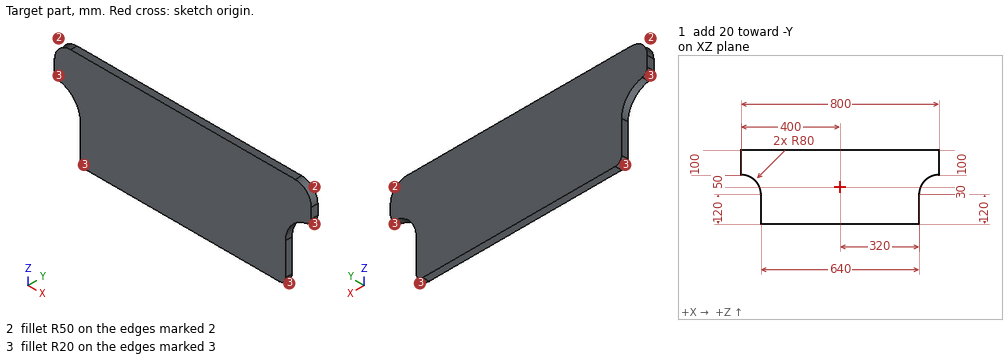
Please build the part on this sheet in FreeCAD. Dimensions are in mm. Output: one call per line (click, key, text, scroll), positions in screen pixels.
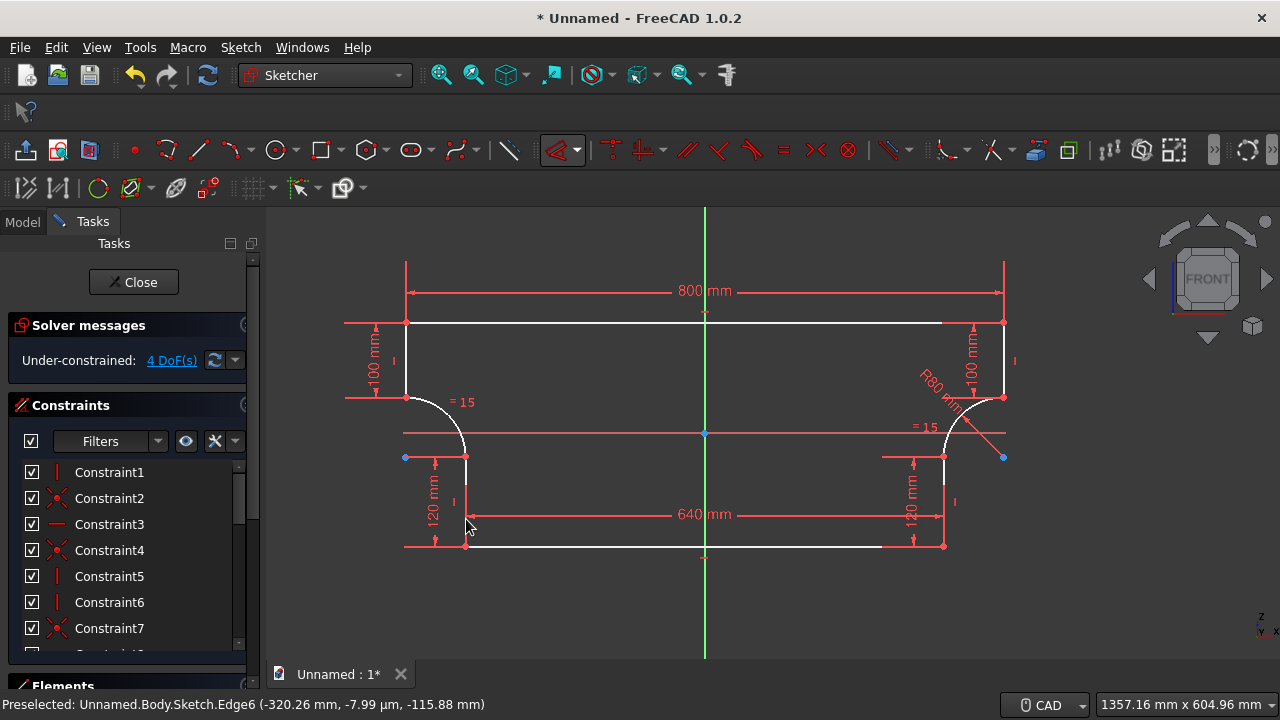
click(406, 398)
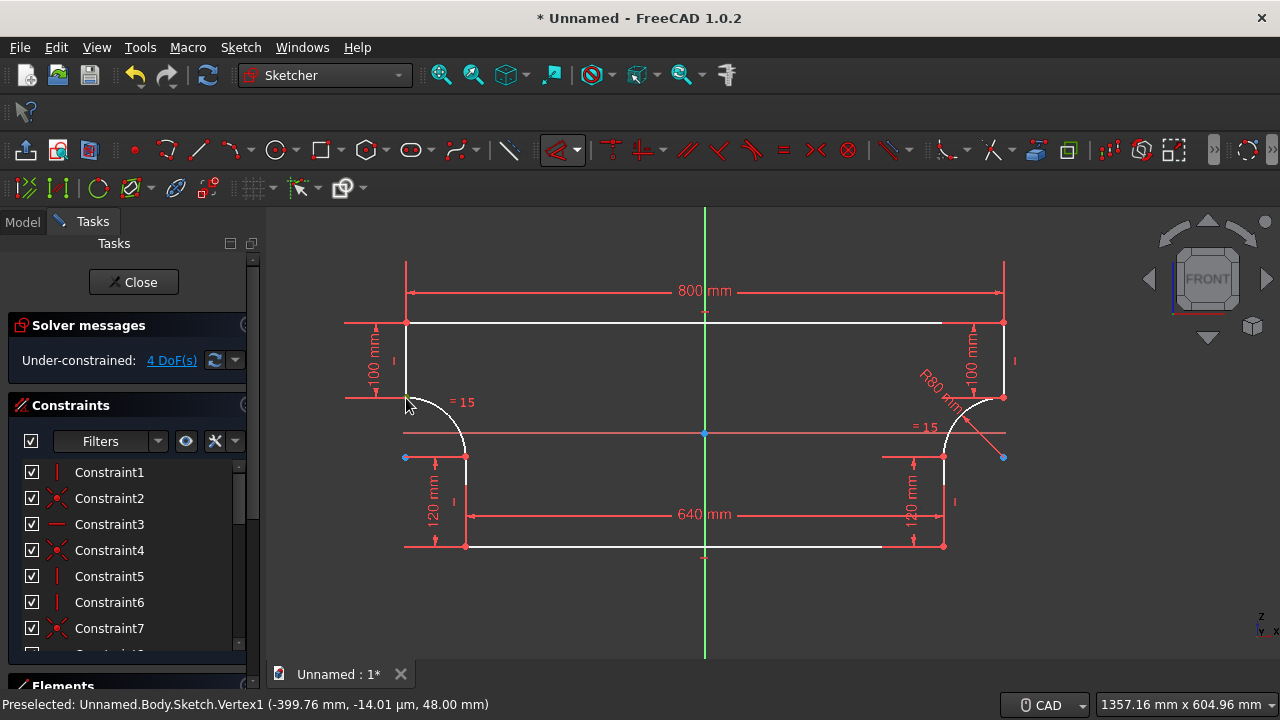
key(i)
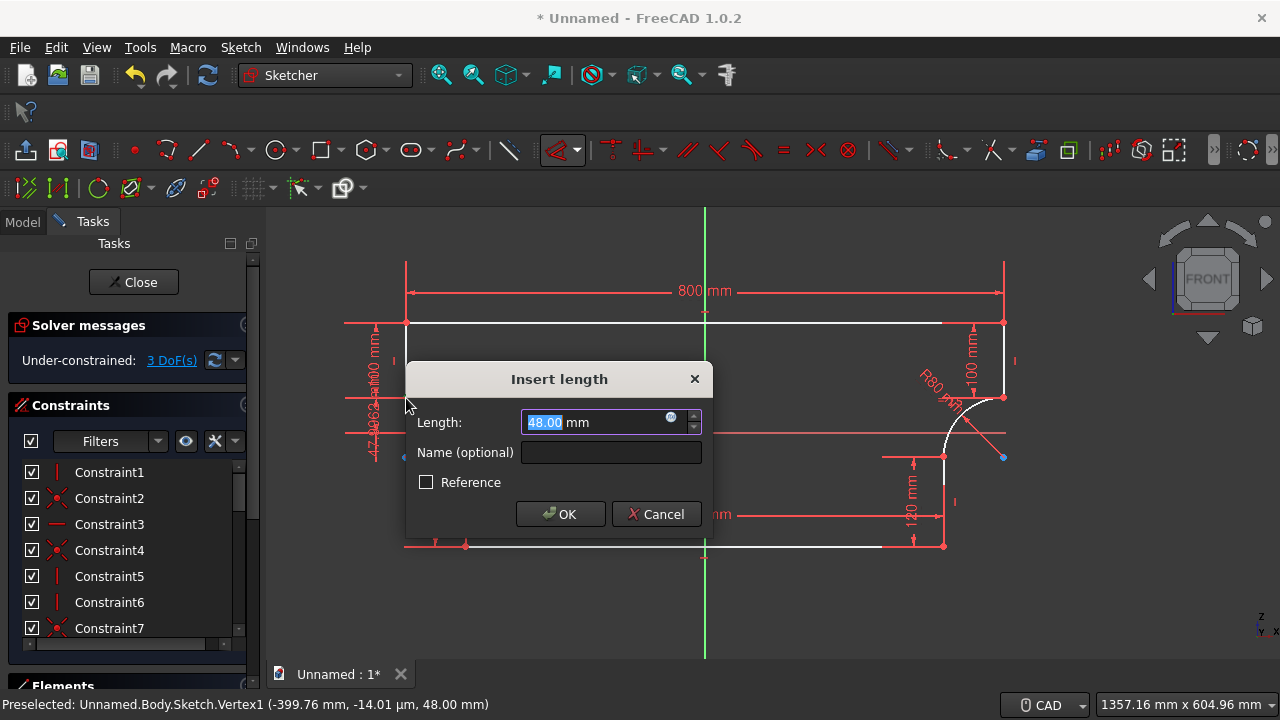
text(50)
key(Return)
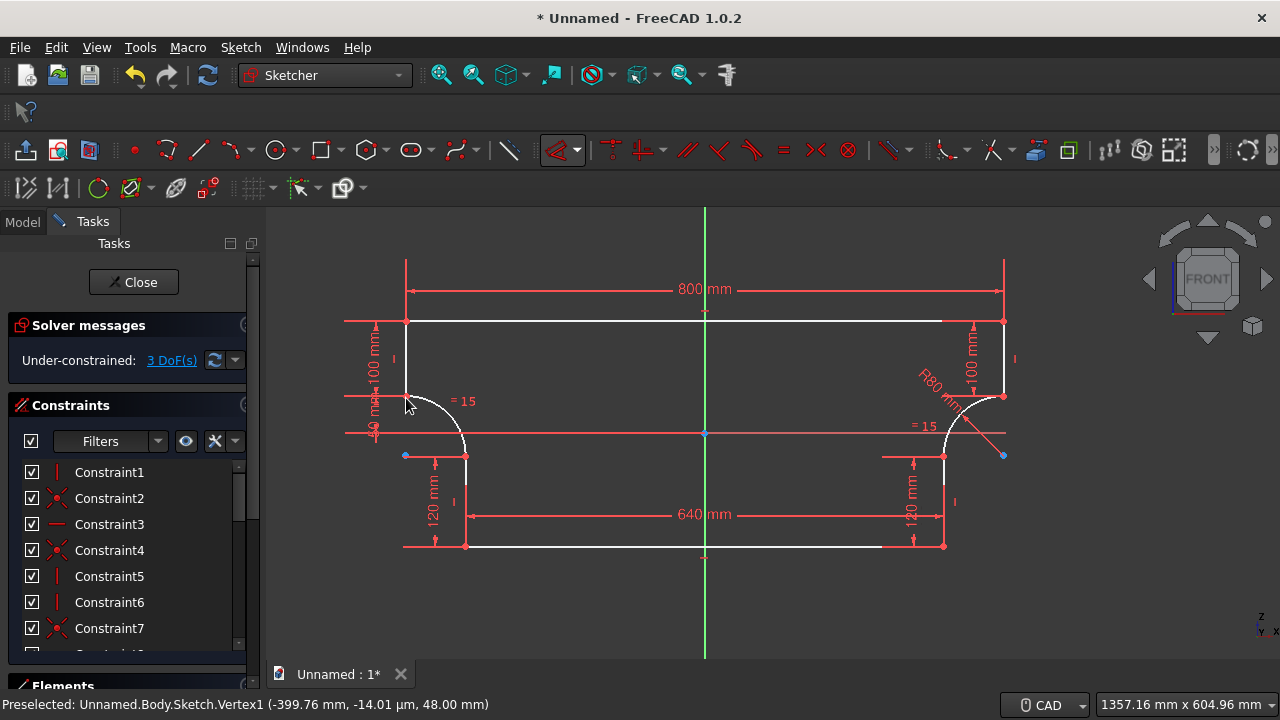
scroll(944, 457, up, 3)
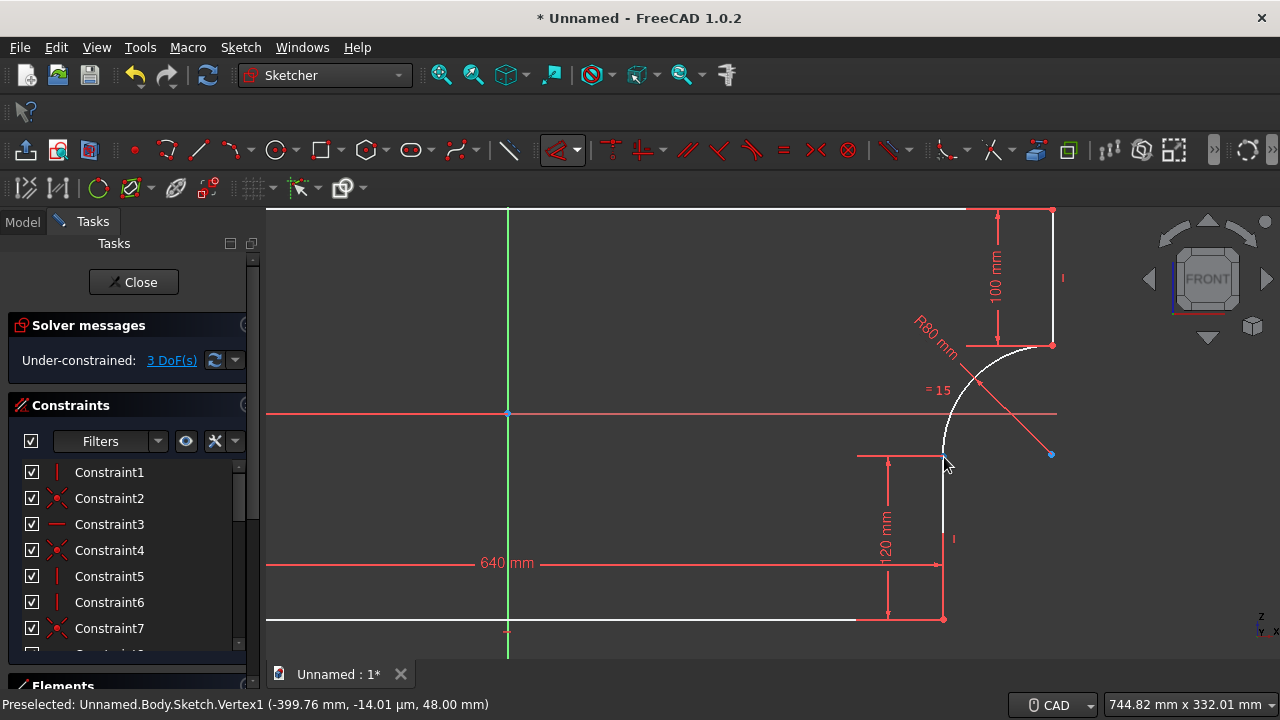
click(943, 456)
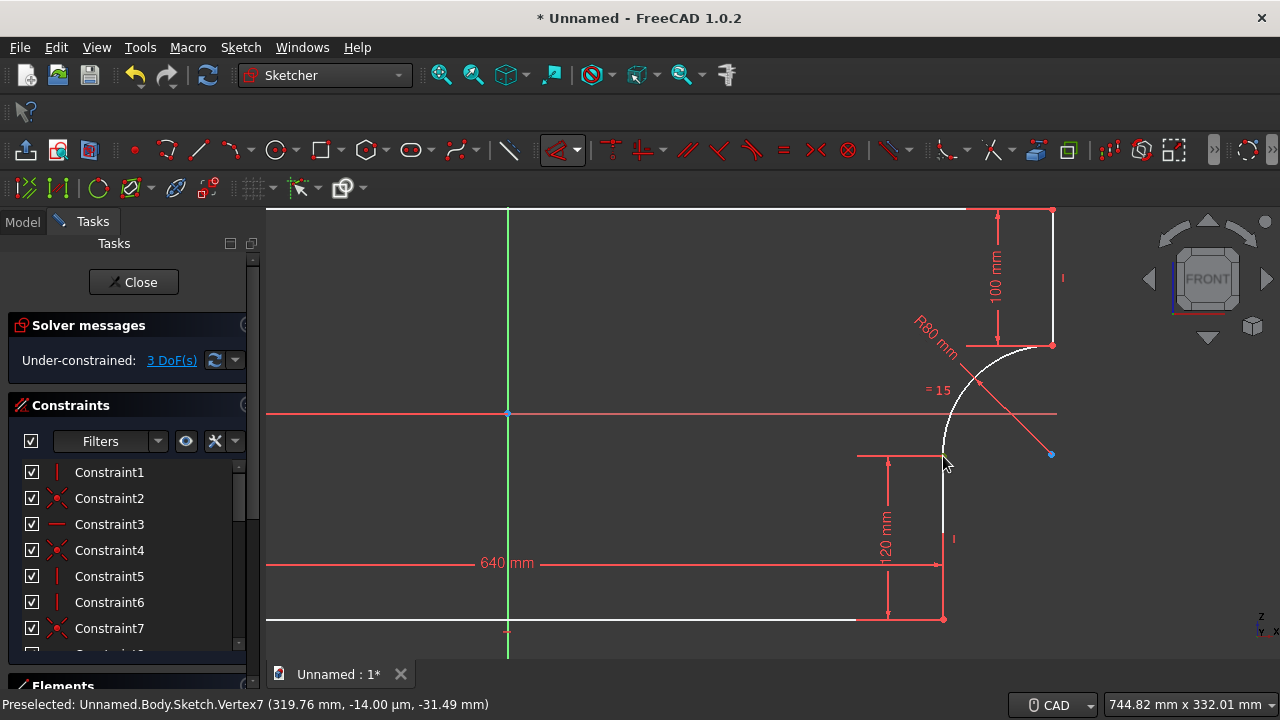
key(i)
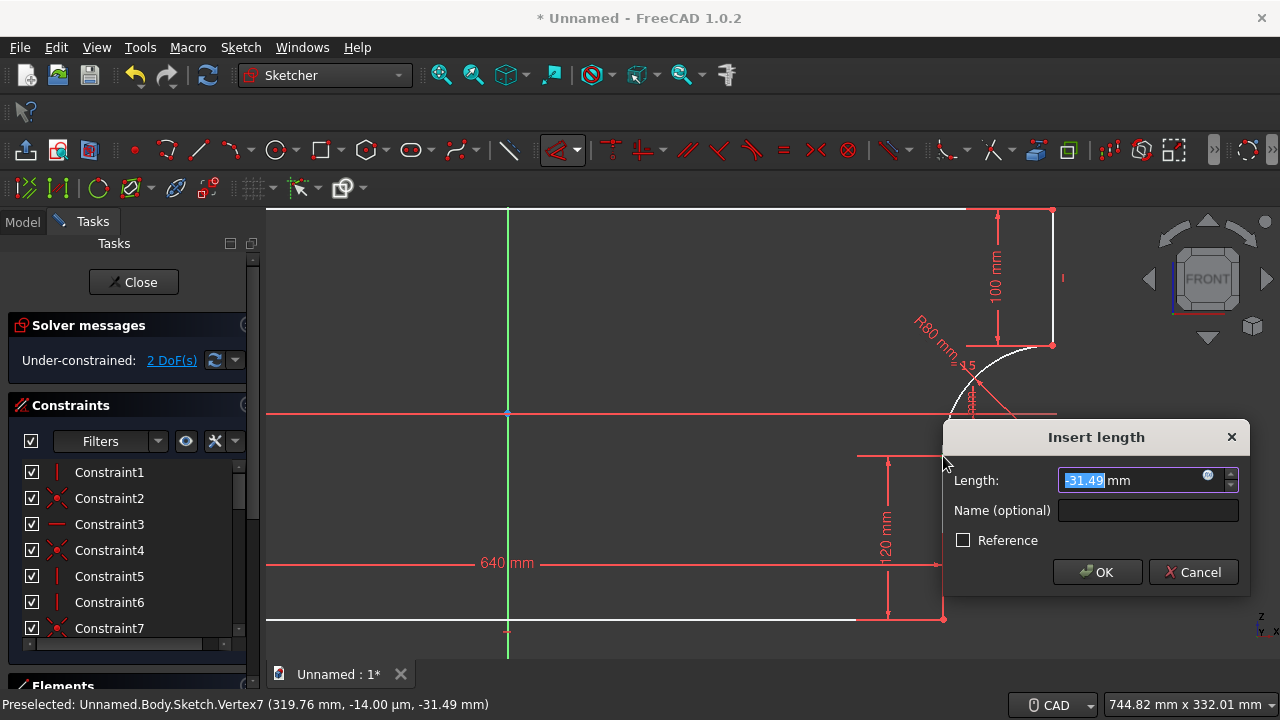
text(-30)
key(Return)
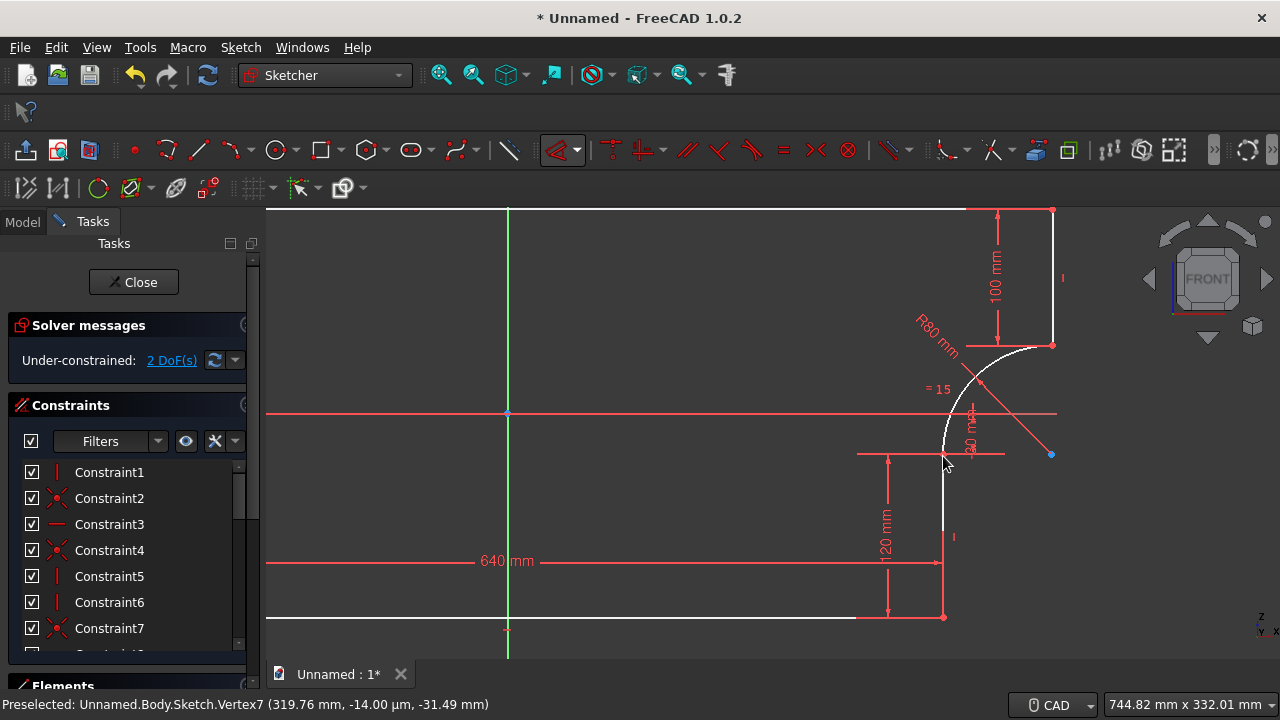
scroll(944, 457, down, 3)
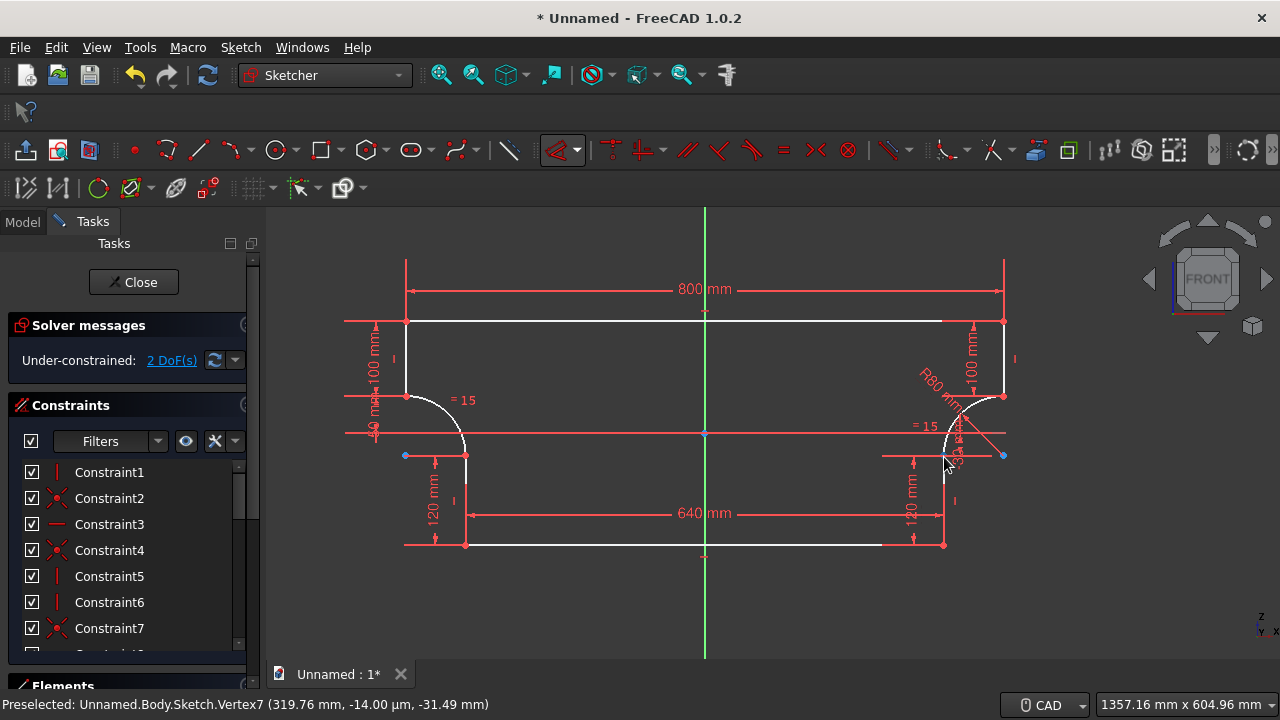
click(406, 396)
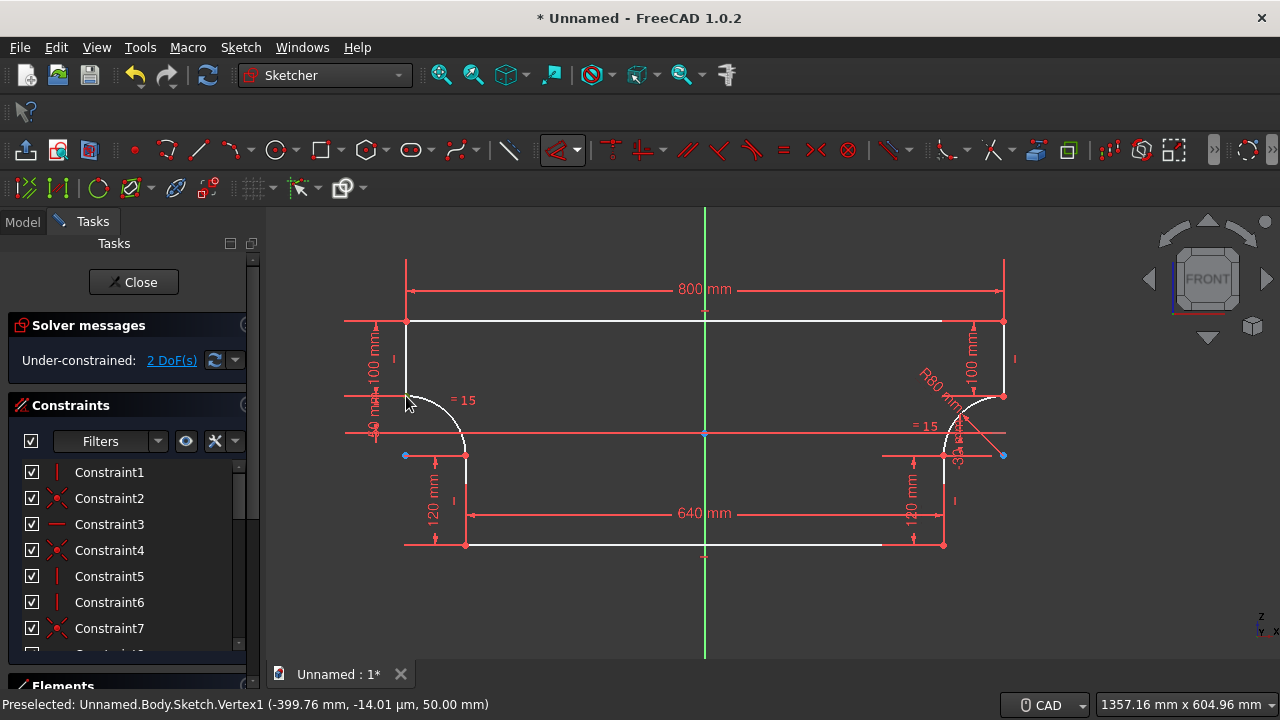
click(580, 150)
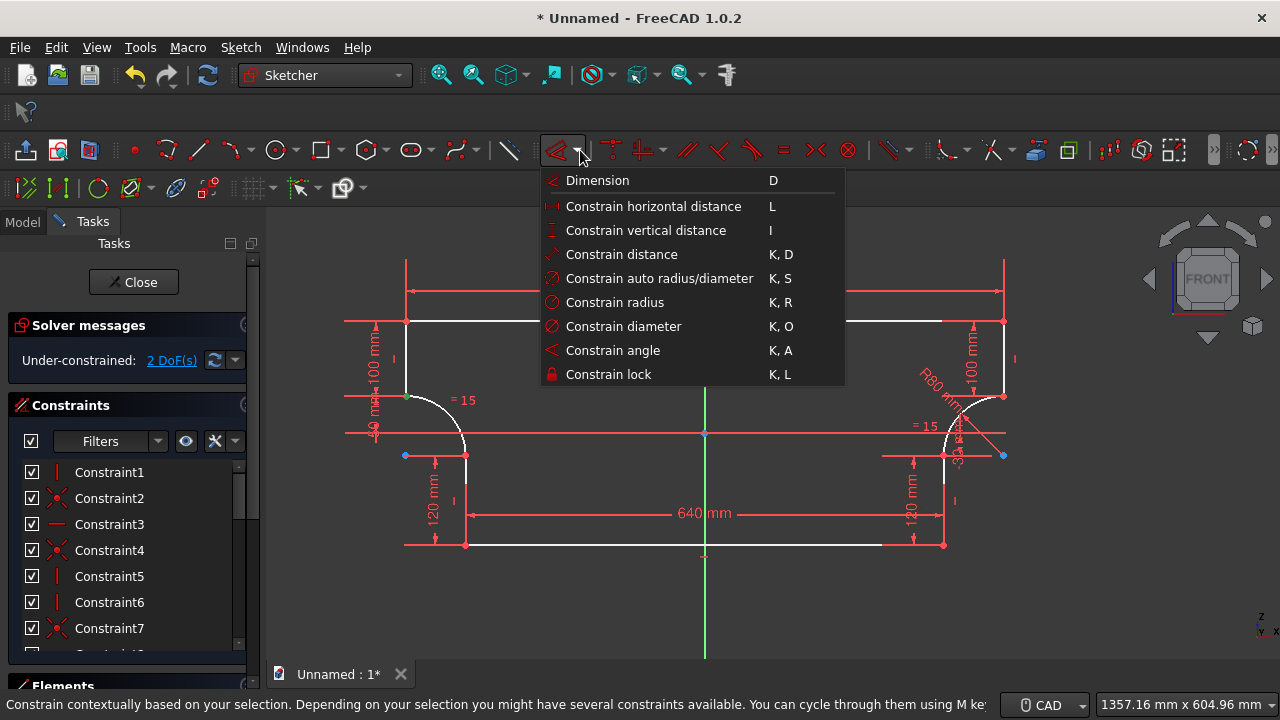
click(693, 206)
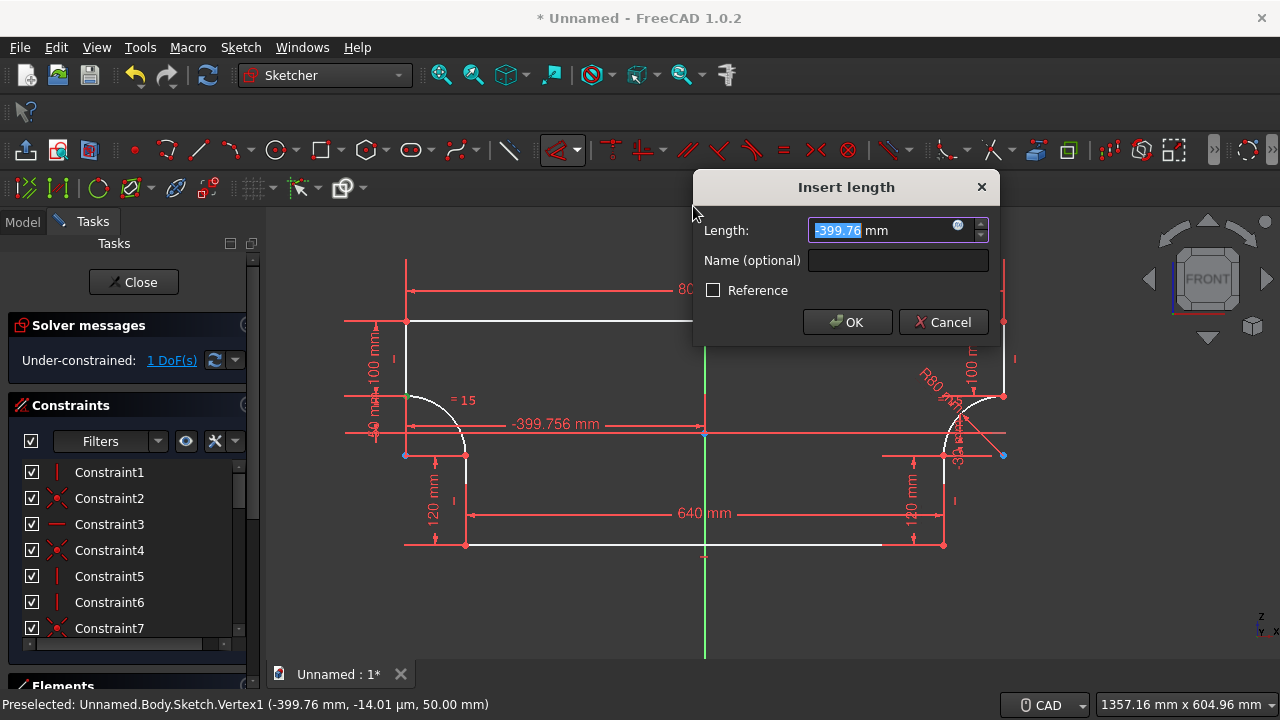
text(-400)
key(Return)